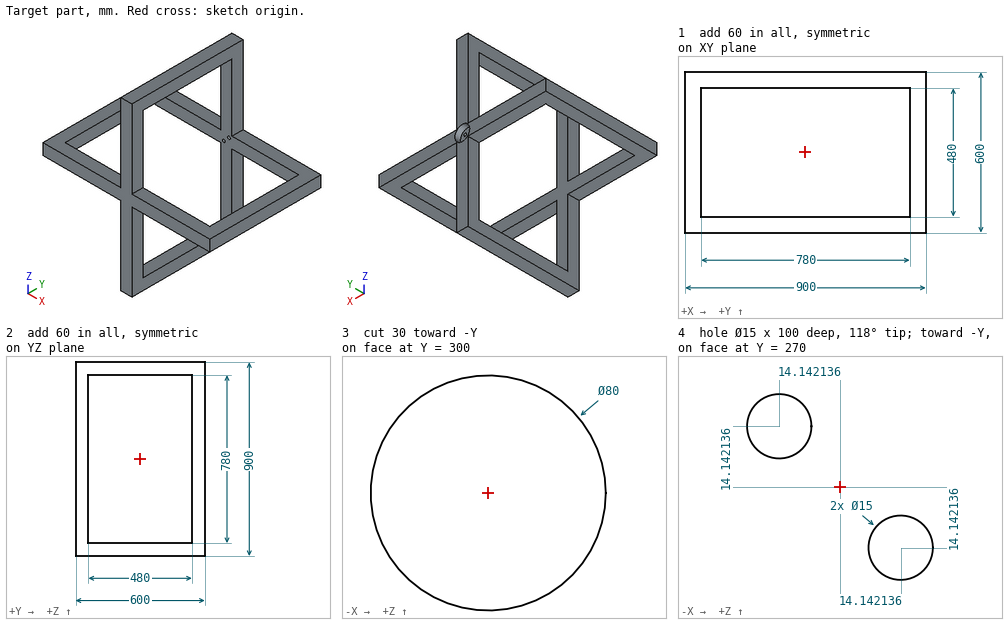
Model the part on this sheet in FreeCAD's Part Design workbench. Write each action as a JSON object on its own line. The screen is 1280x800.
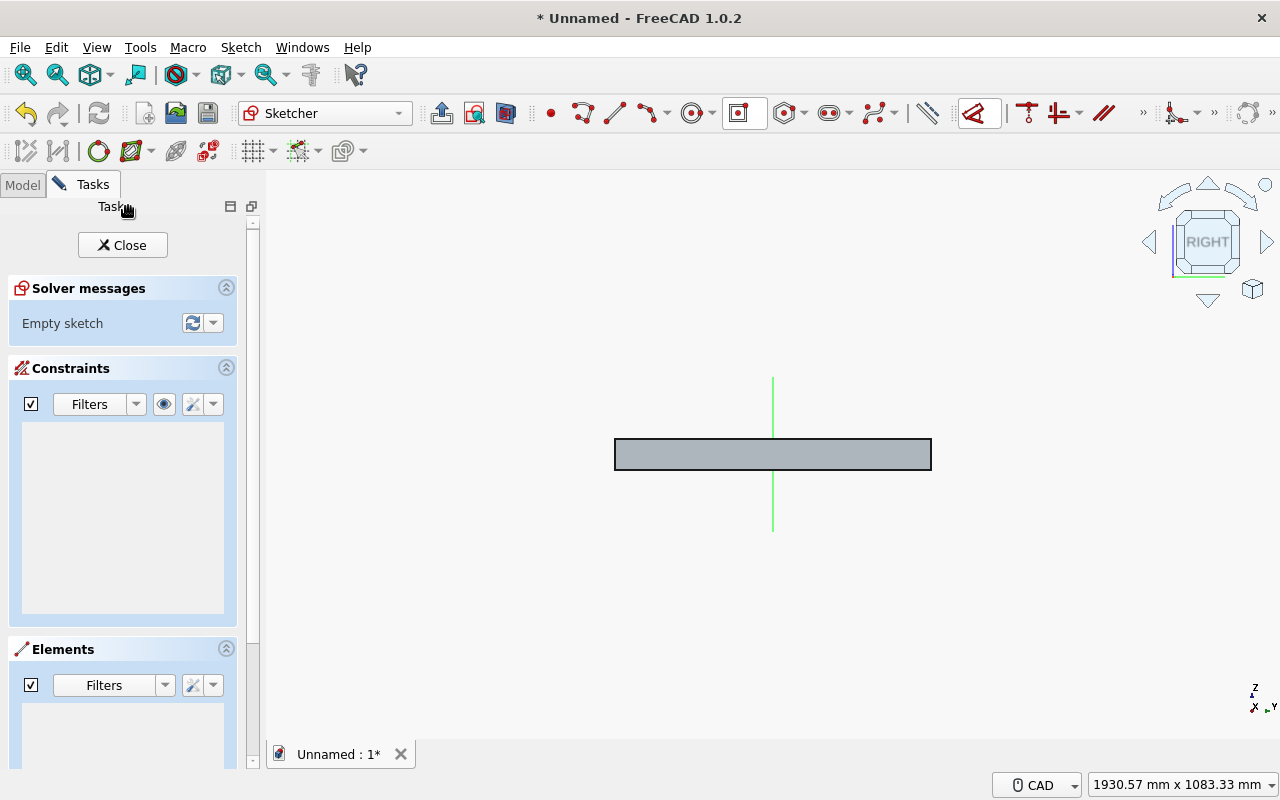
{"action": "left_click", "coordinate": [506, 114]}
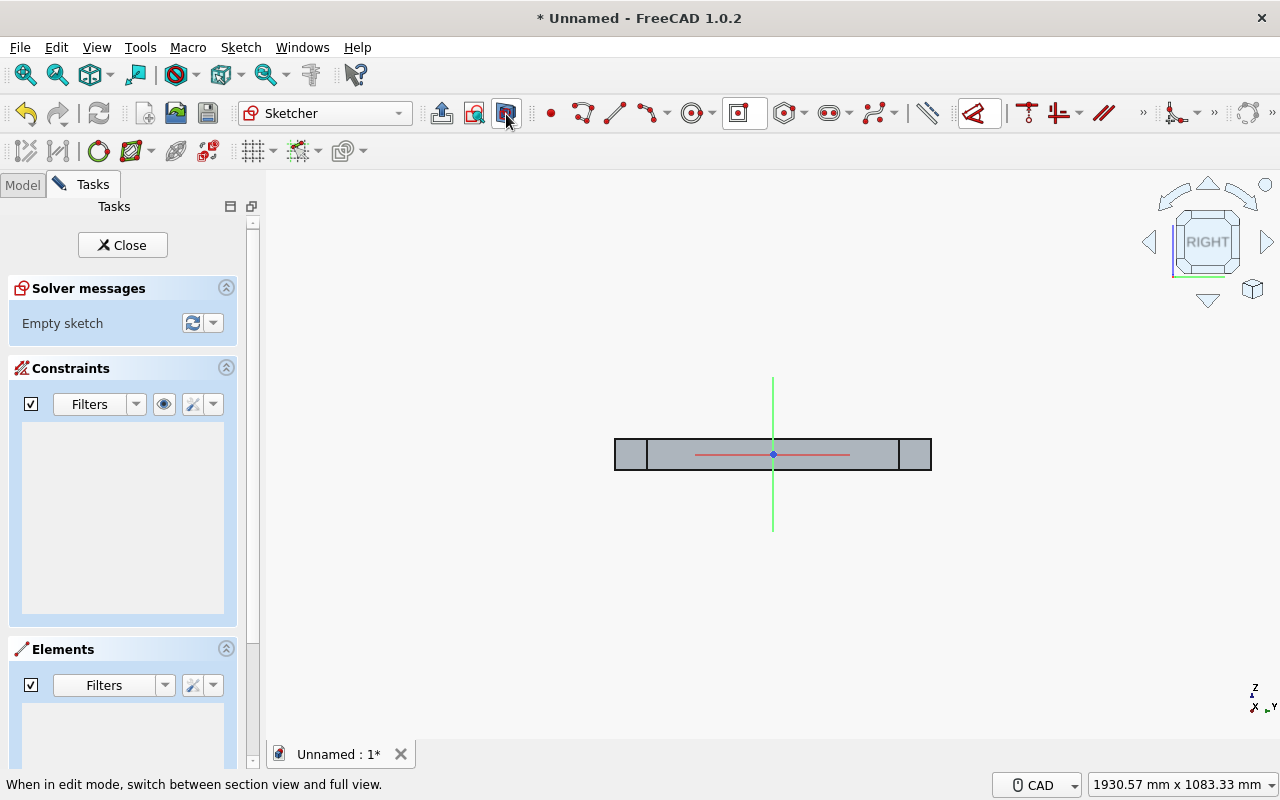
{"action": "scroll", "coordinate": [395, 455], "scroll_direction": "down", "scroll_amount": 1}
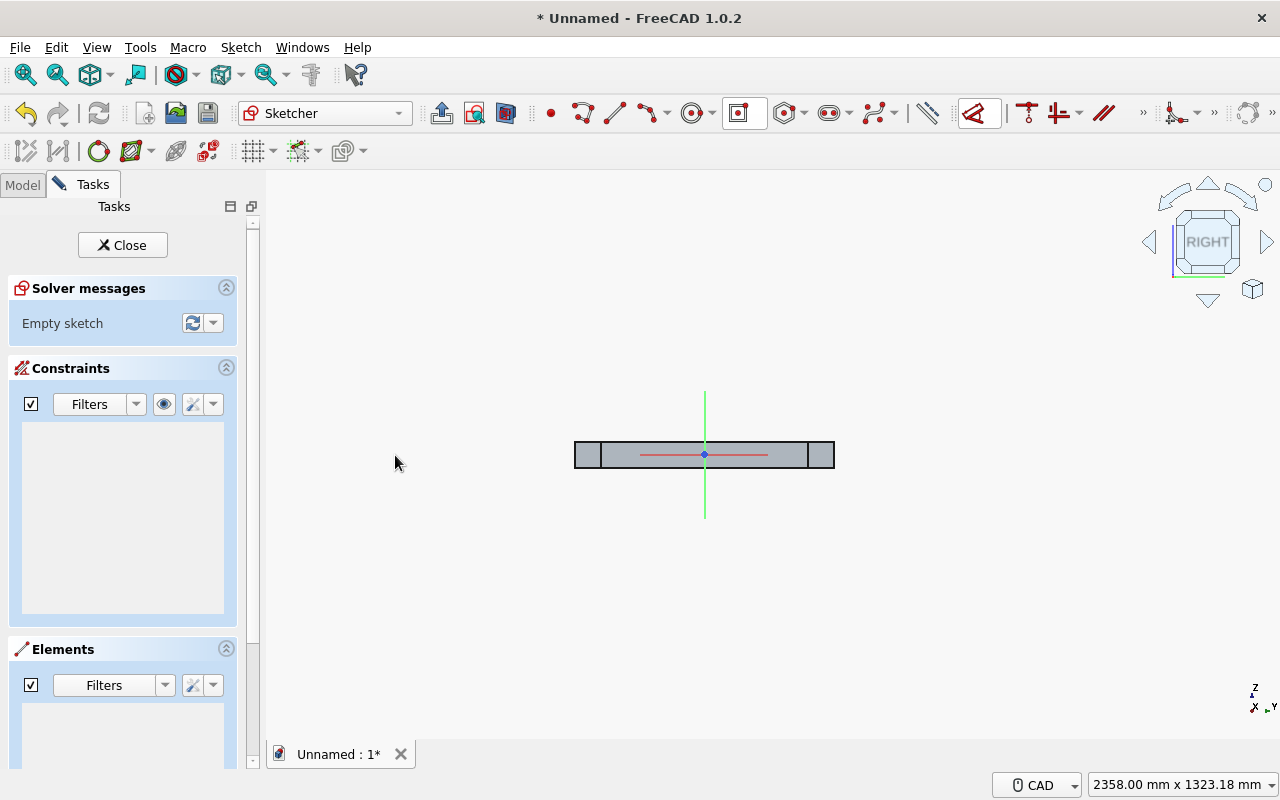
{"action": "left_click", "coordinate": [738, 114]}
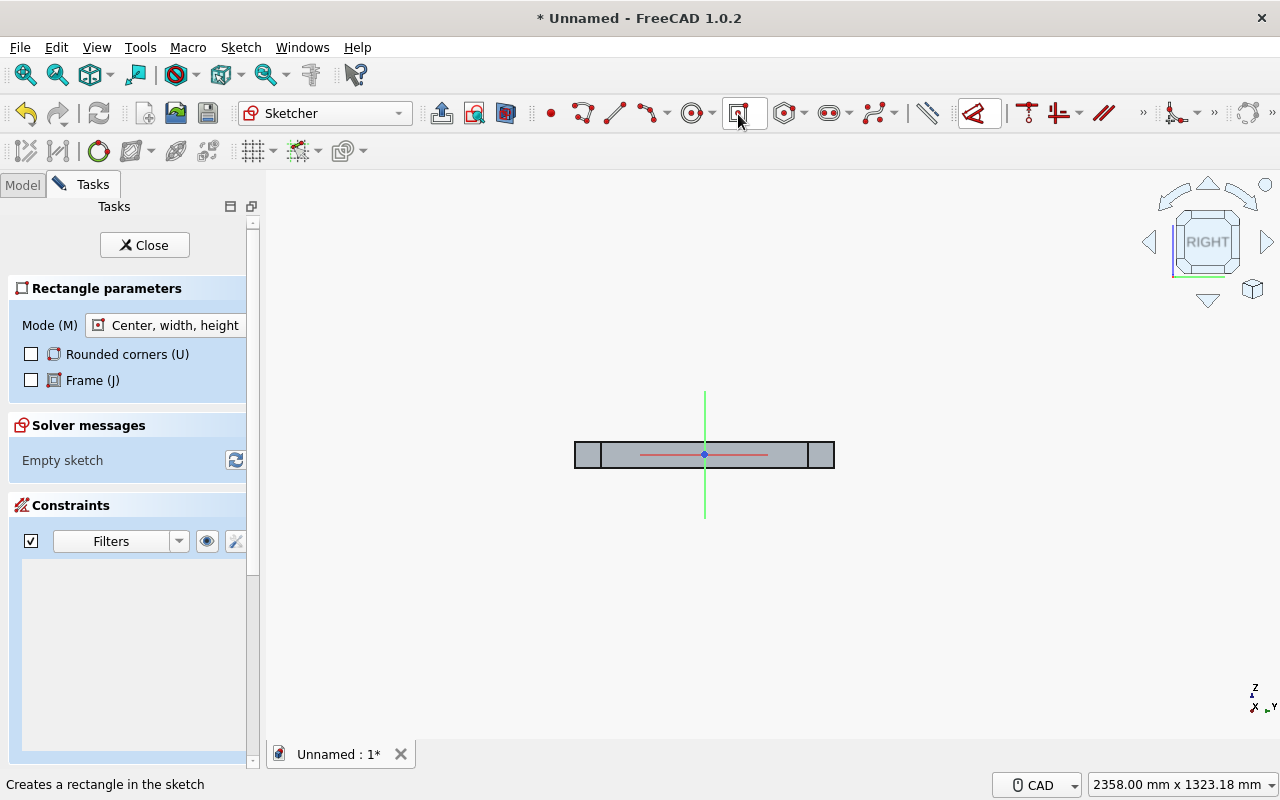
{"action": "left_click", "coordinate": [705, 455]}
{"action": "mouse_move", "coordinate": [834, 261]}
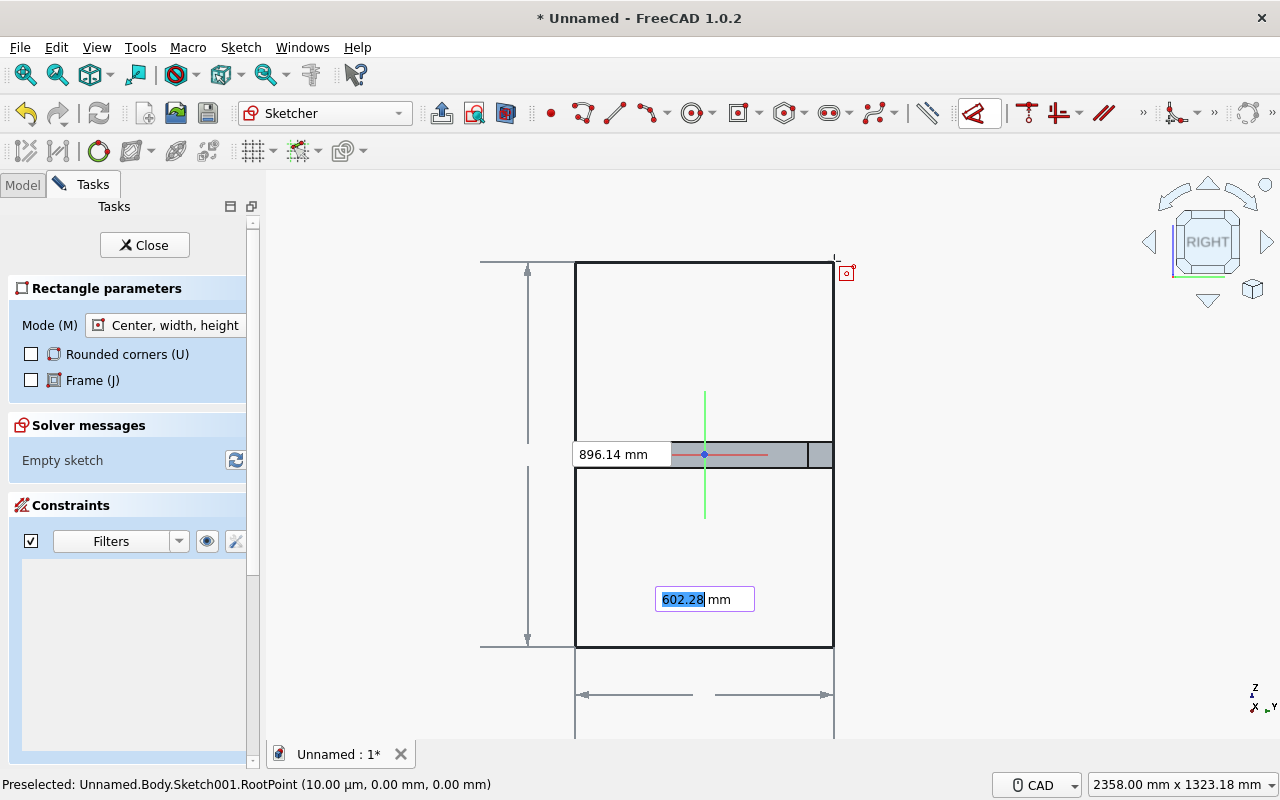
{"action": "type", "text": "600"}
{"action": "key", "text": "Tab"}
{"action": "type", "text": "900"}
{"action": "key", "text": "Return"}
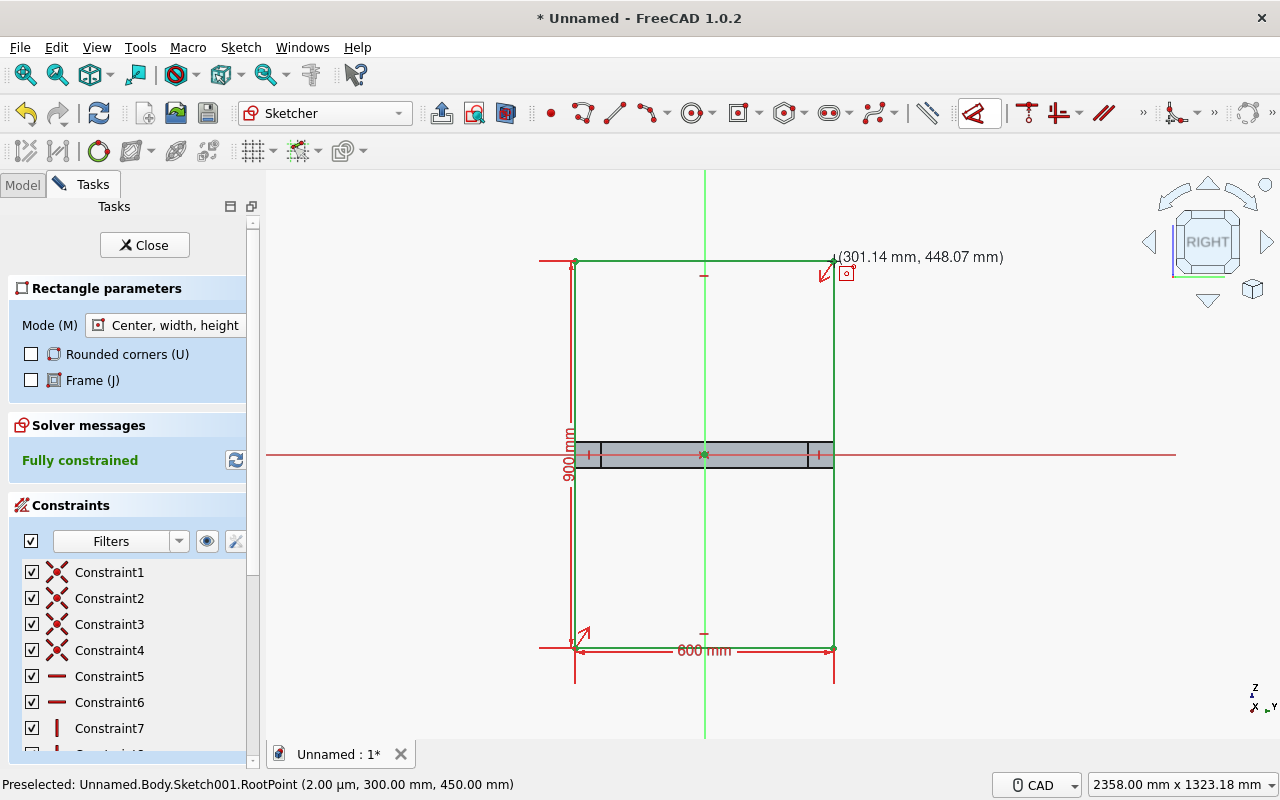
{"action": "left_click", "coordinate": [705, 455]}
{"action": "mouse_move", "coordinate": [808, 287]}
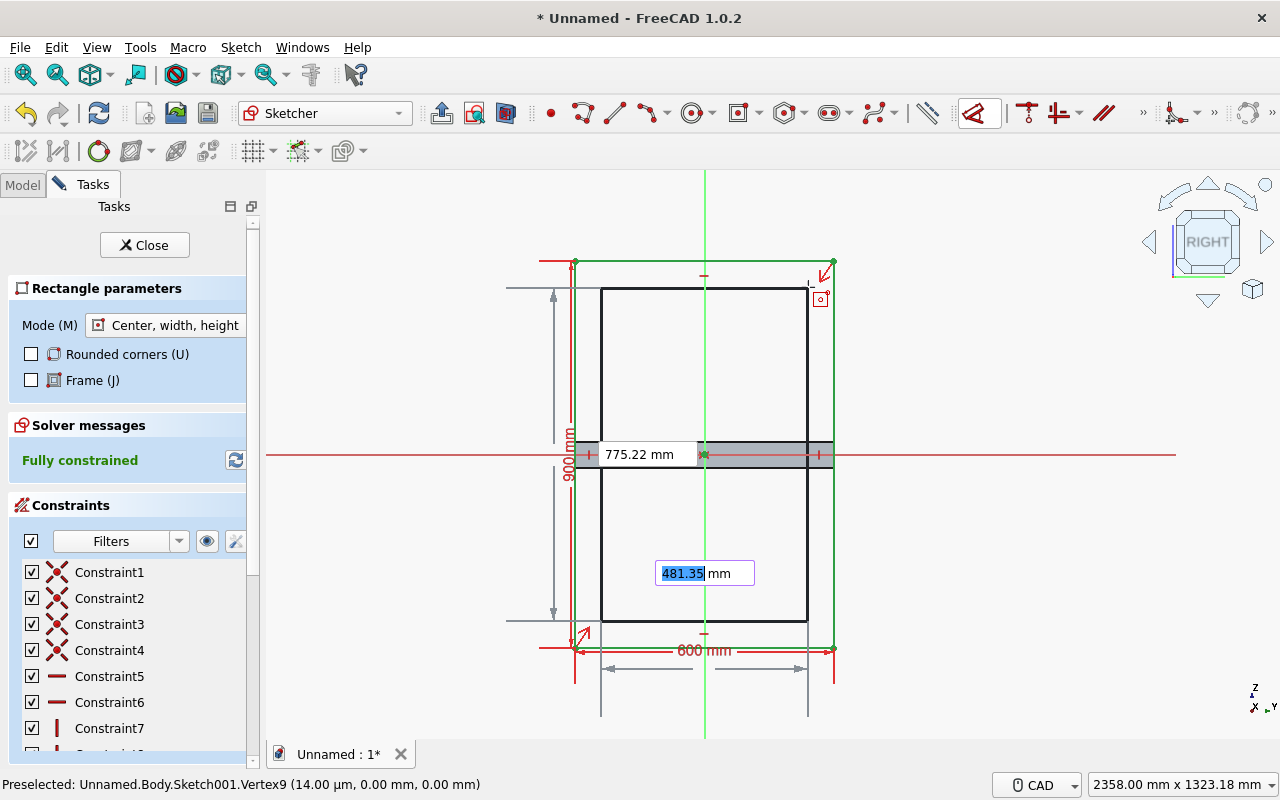
{"action": "type", "text": "480"}
{"action": "key", "text": "Tab"}
{"action": "type", "text": "780"}
{"action": "key", "text": "Return"}
{"action": "key", "text": "Escape"}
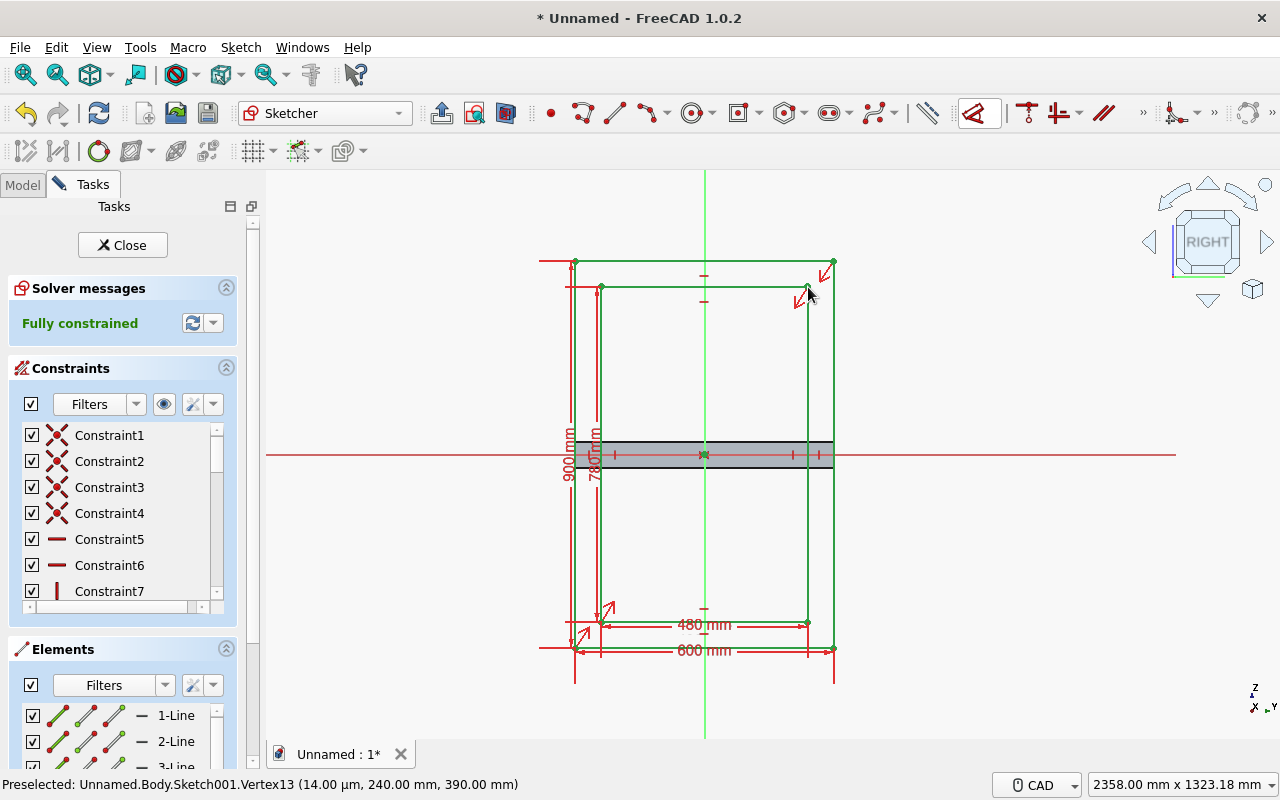
{"action": "left_click", "coordinate": [123, 245]}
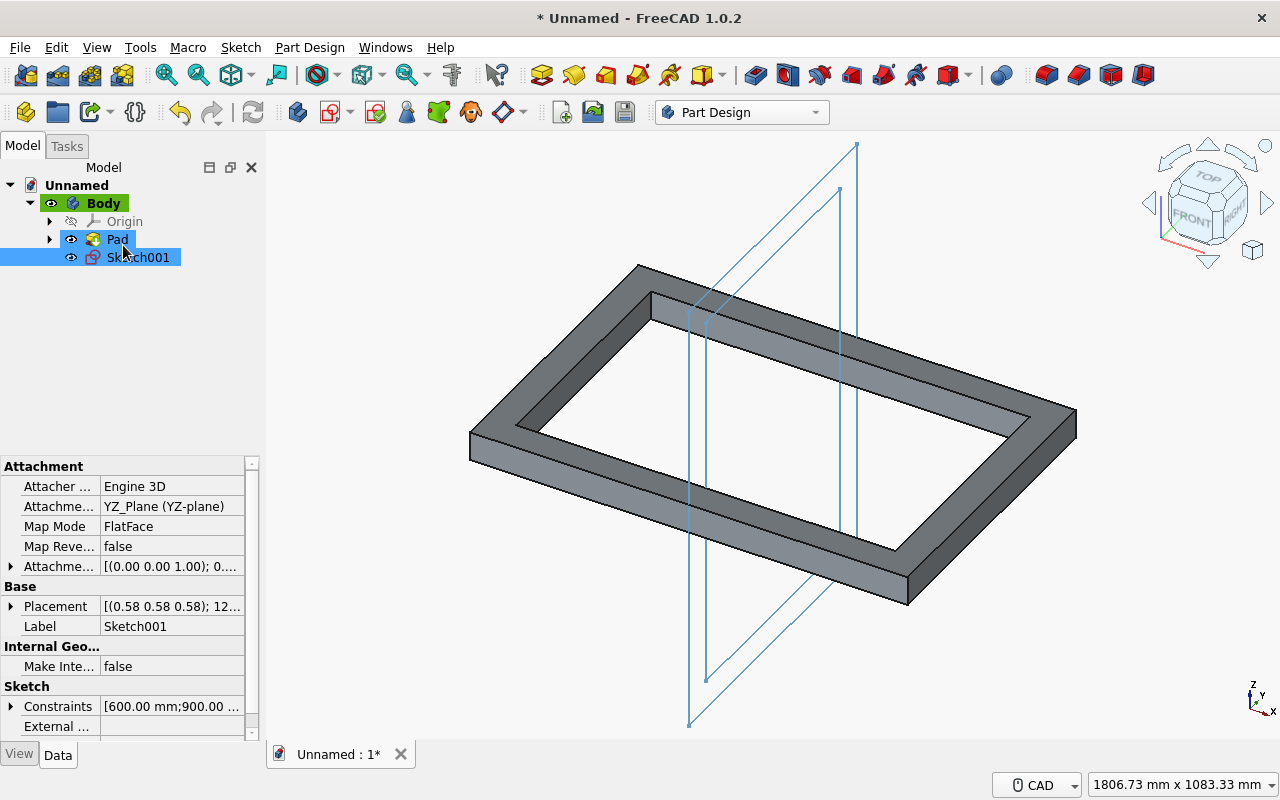
{"action": "left_click", "coordinate": [542, 76]}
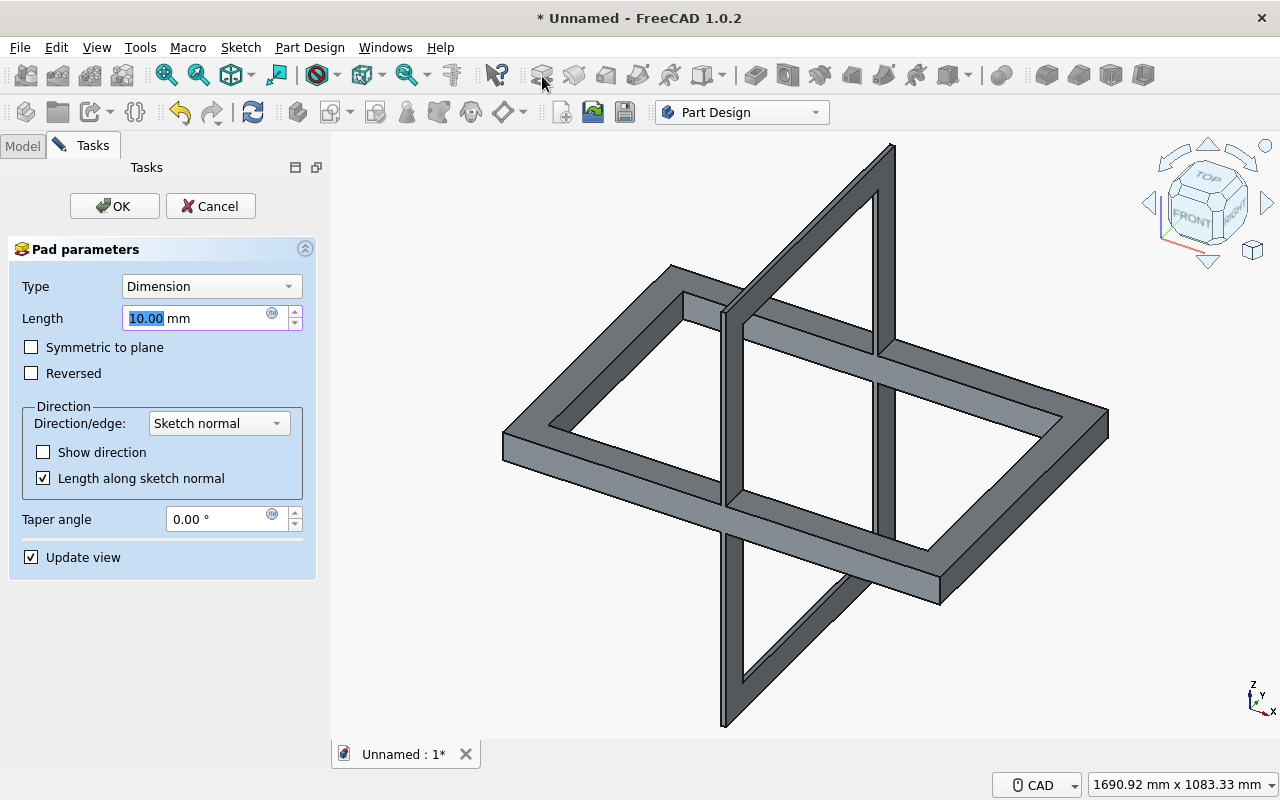
{"action": "type", "text": "60"}
{"action": "key", "text": "Tab"}